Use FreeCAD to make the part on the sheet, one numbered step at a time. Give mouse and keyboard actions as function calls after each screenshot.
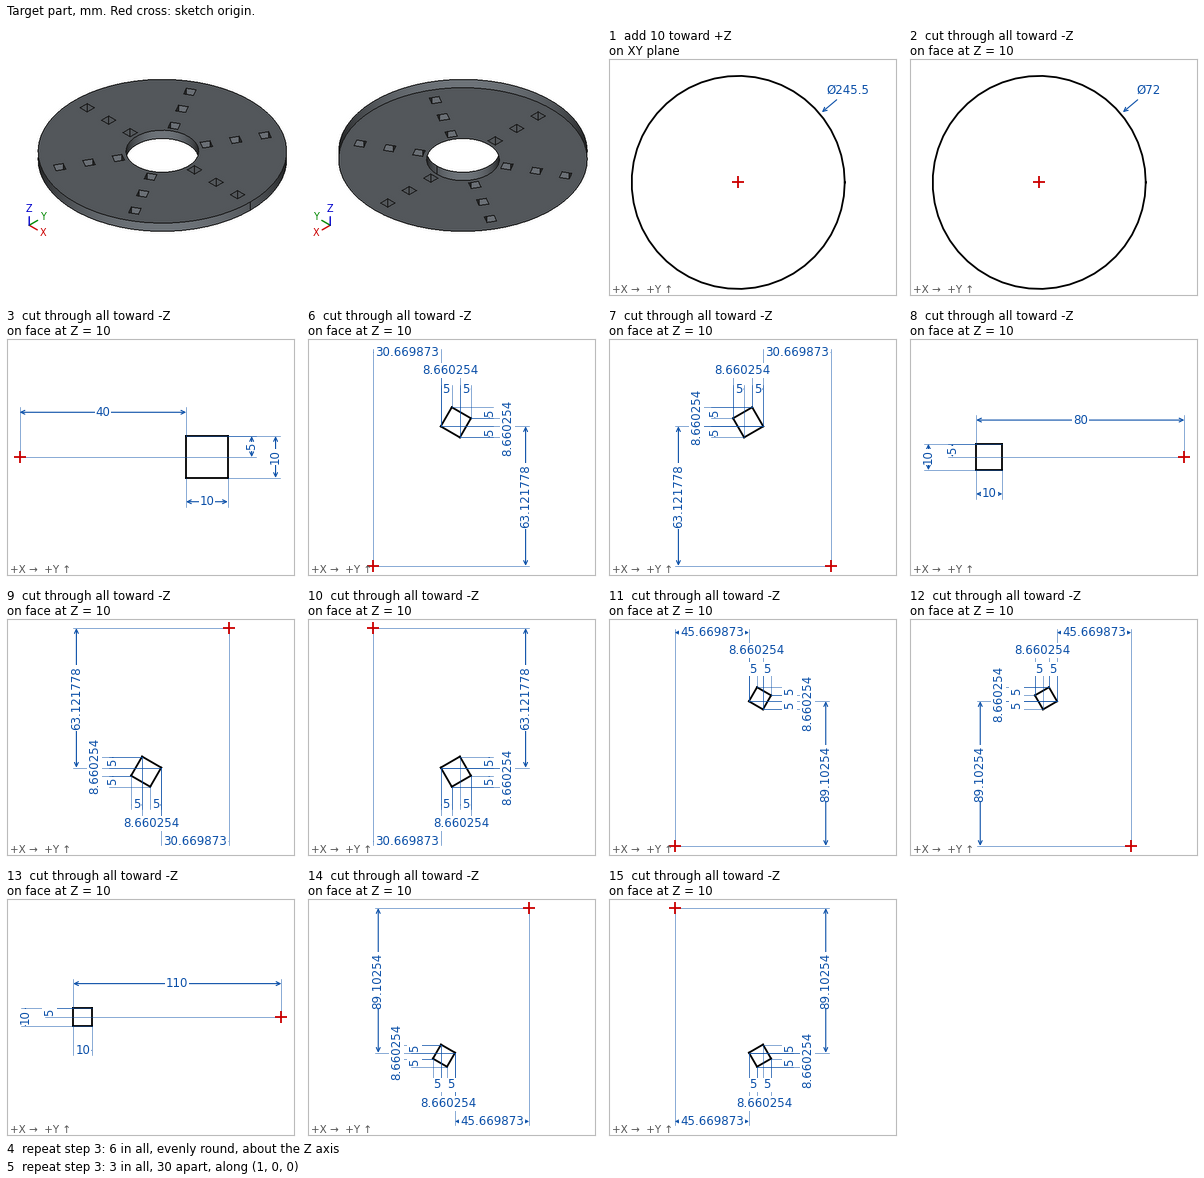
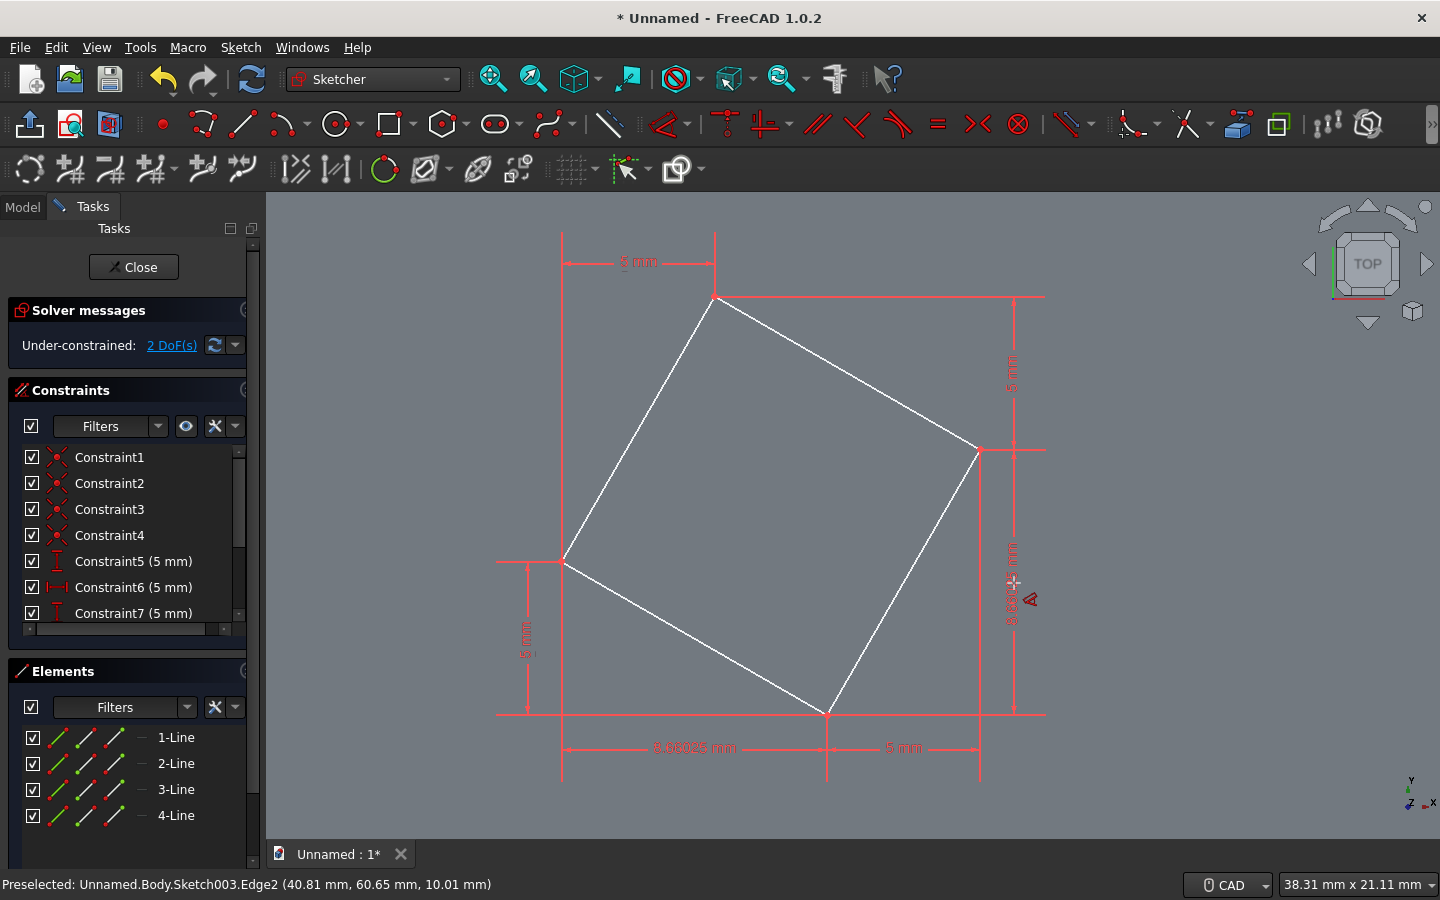
click(562, 562)
click(428, 528)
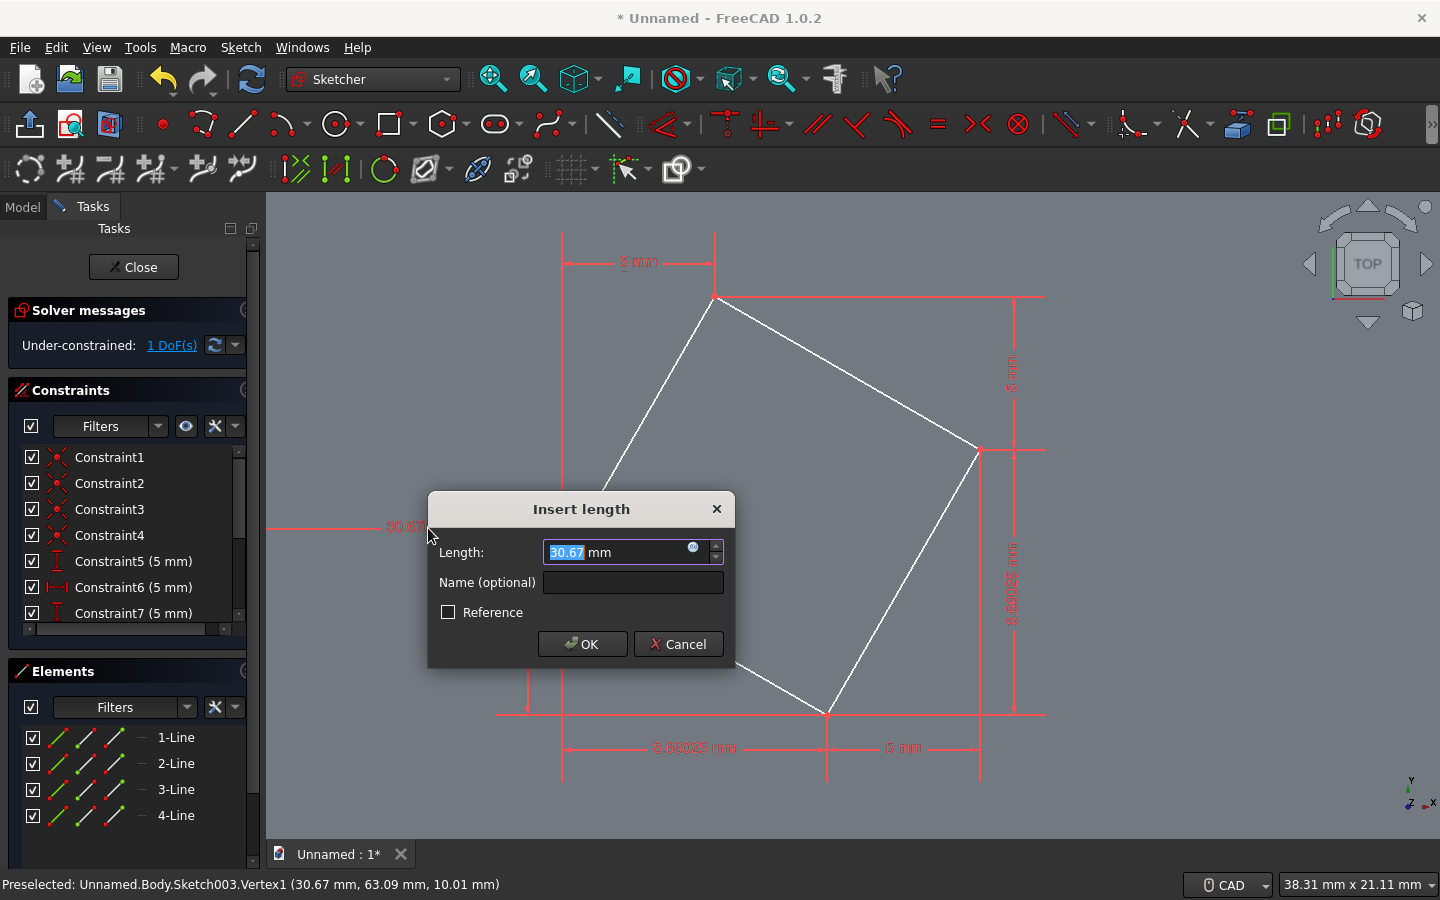
text(30.669873)
key(Return)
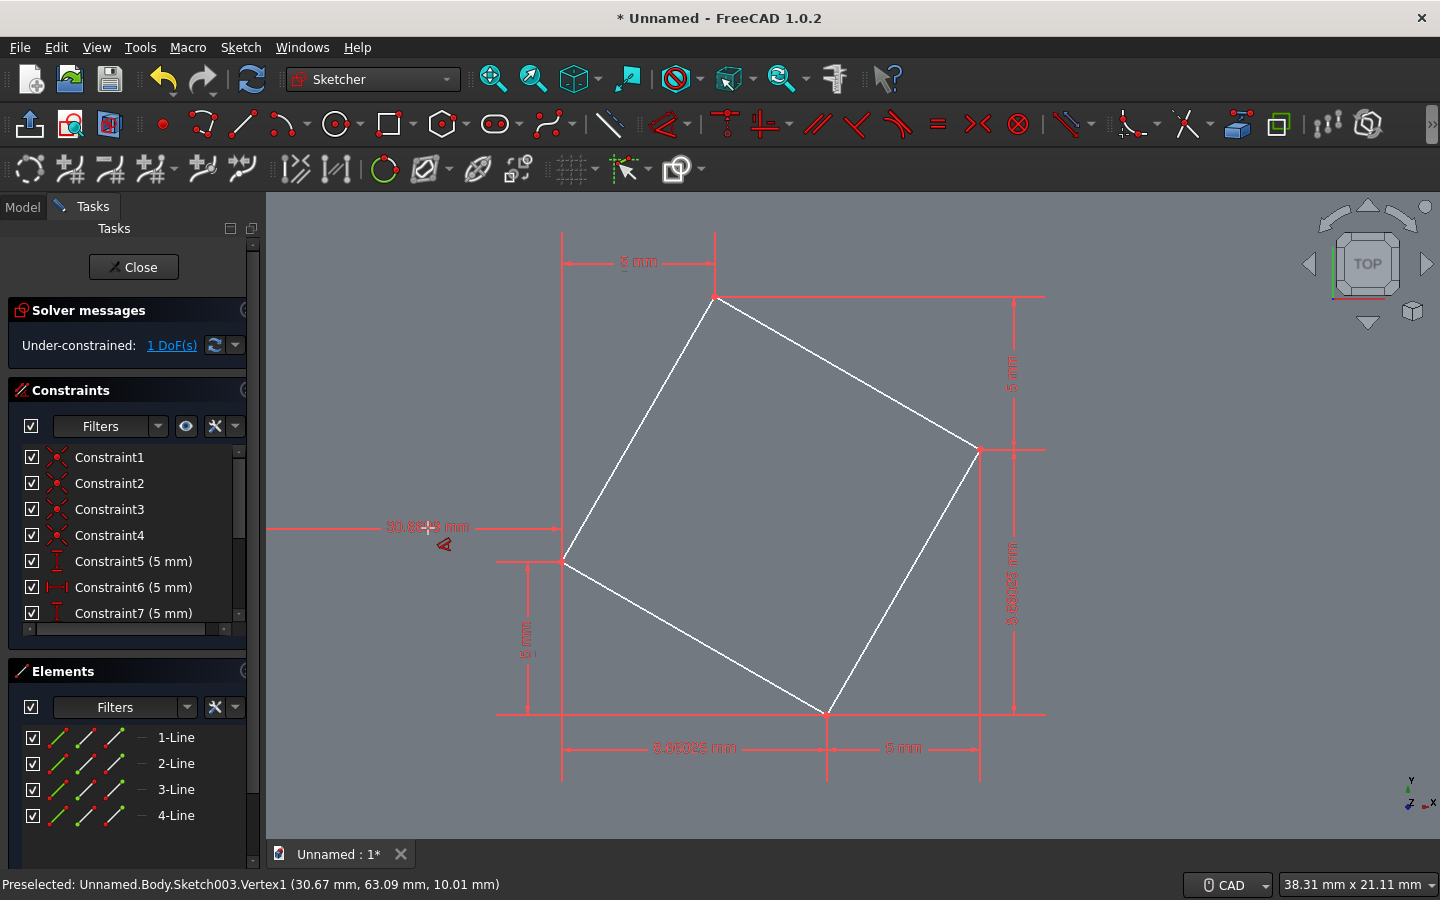
click(562, 562)
click(596, 687)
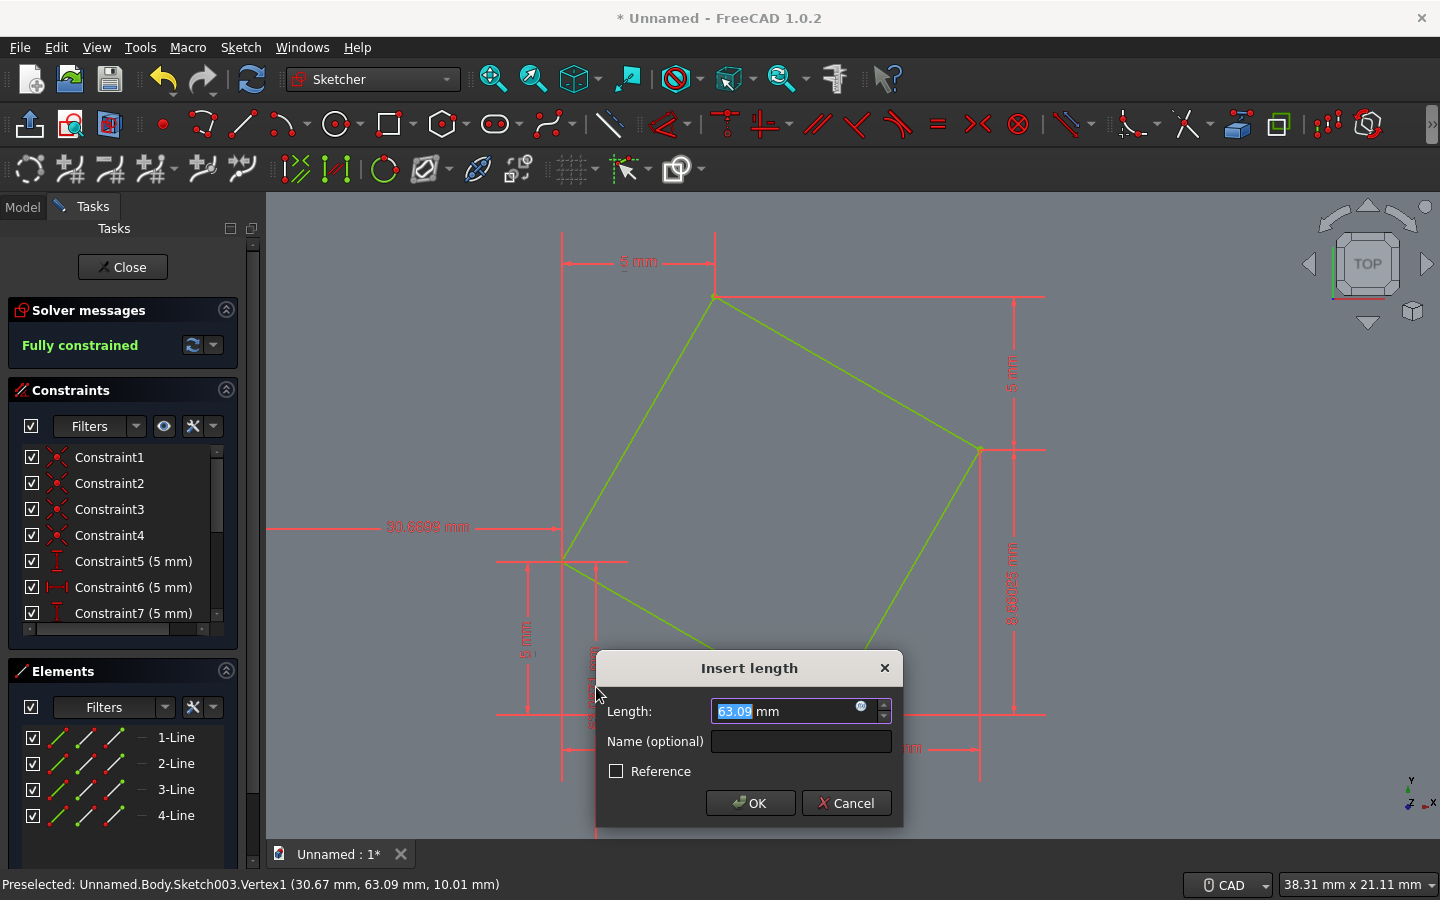
text(63.121778)
key(Return)
key(Escape)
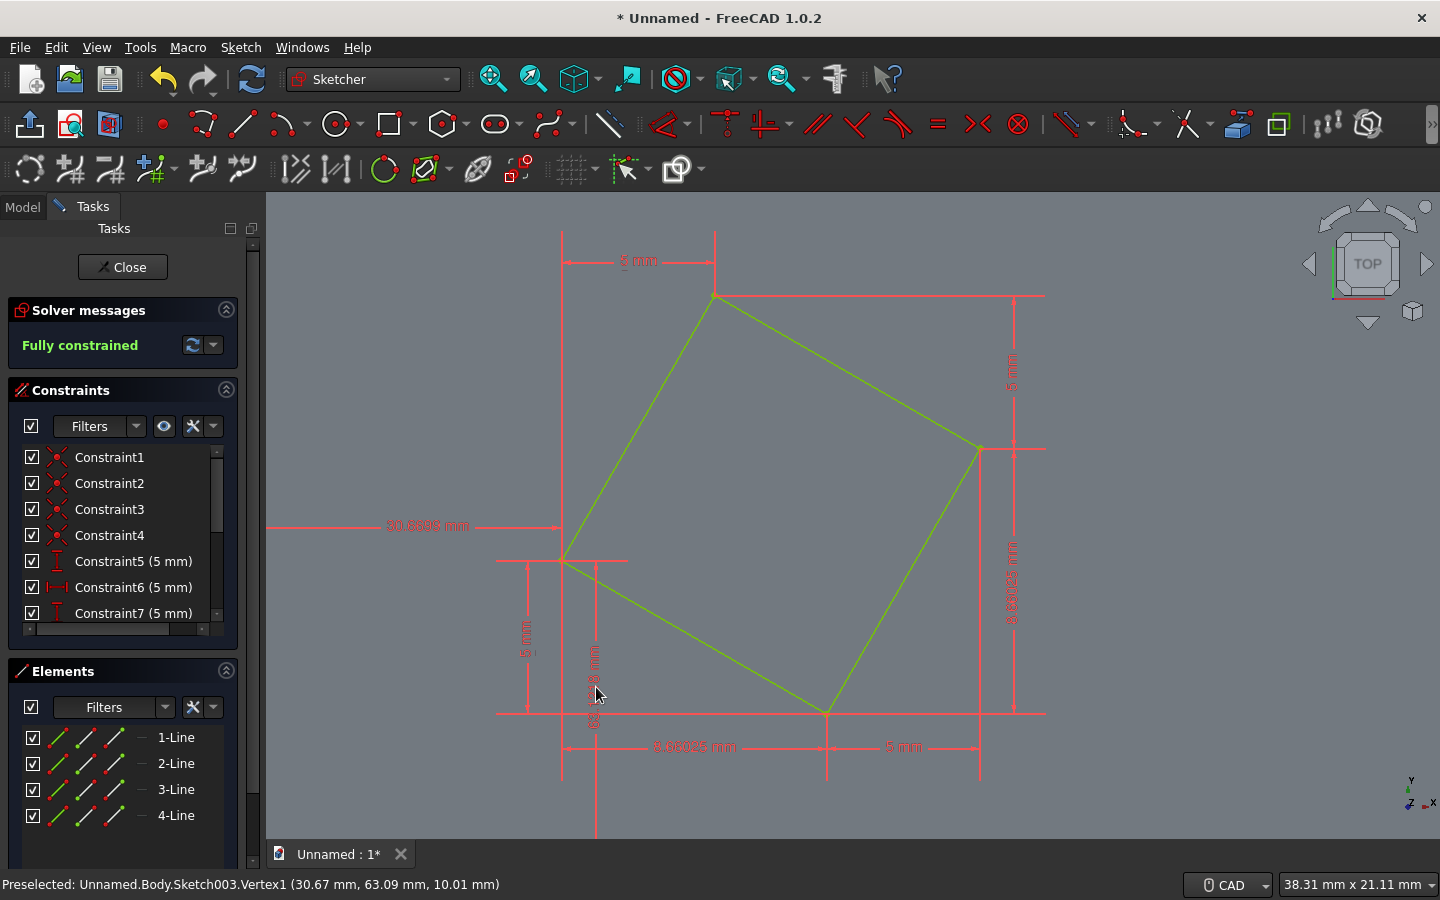
click(123, 267)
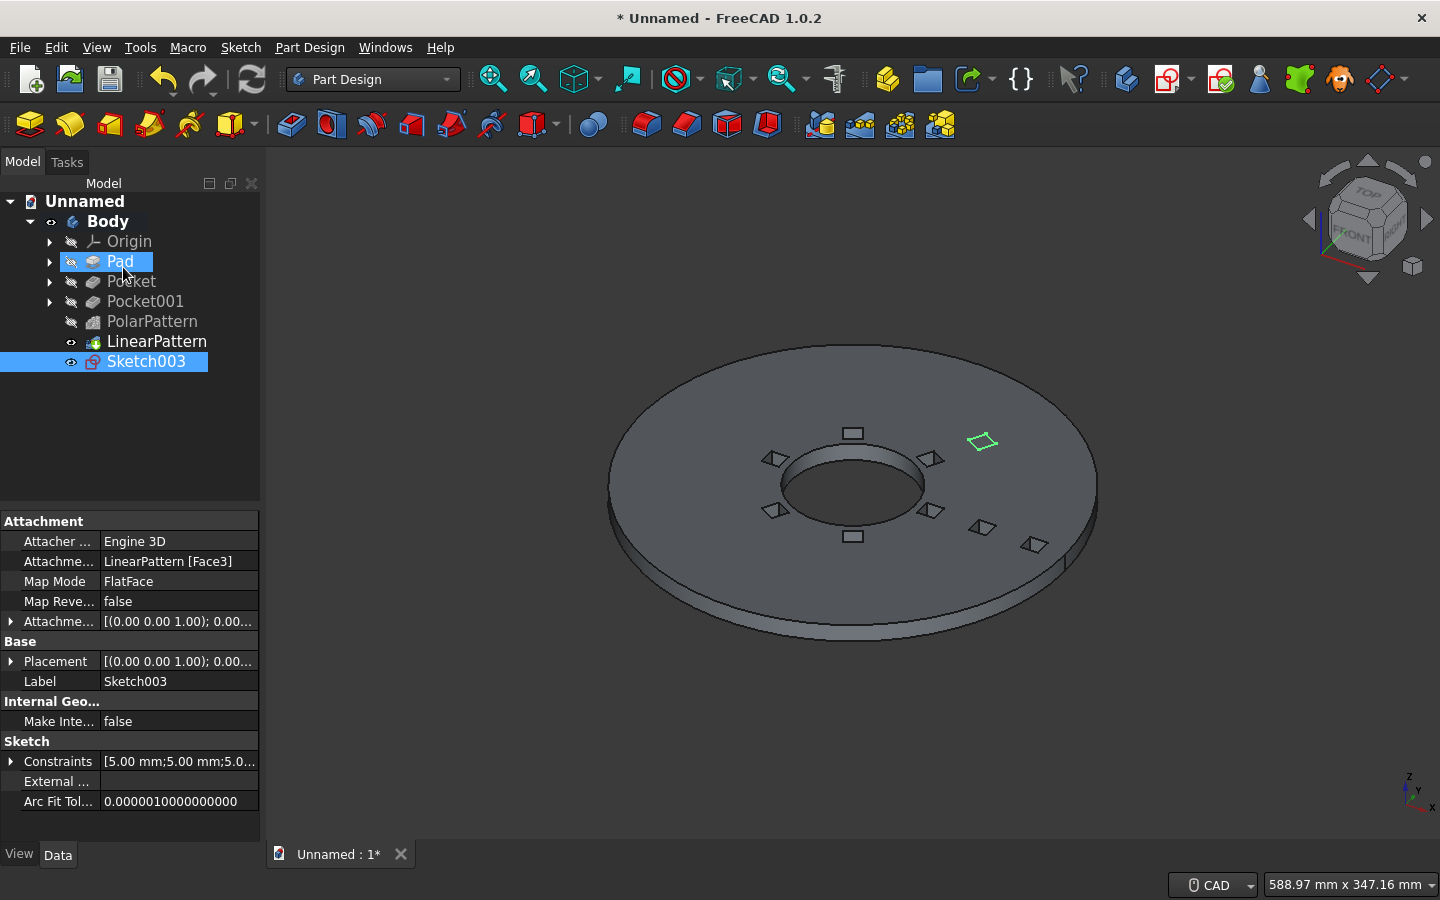
click(292, 124)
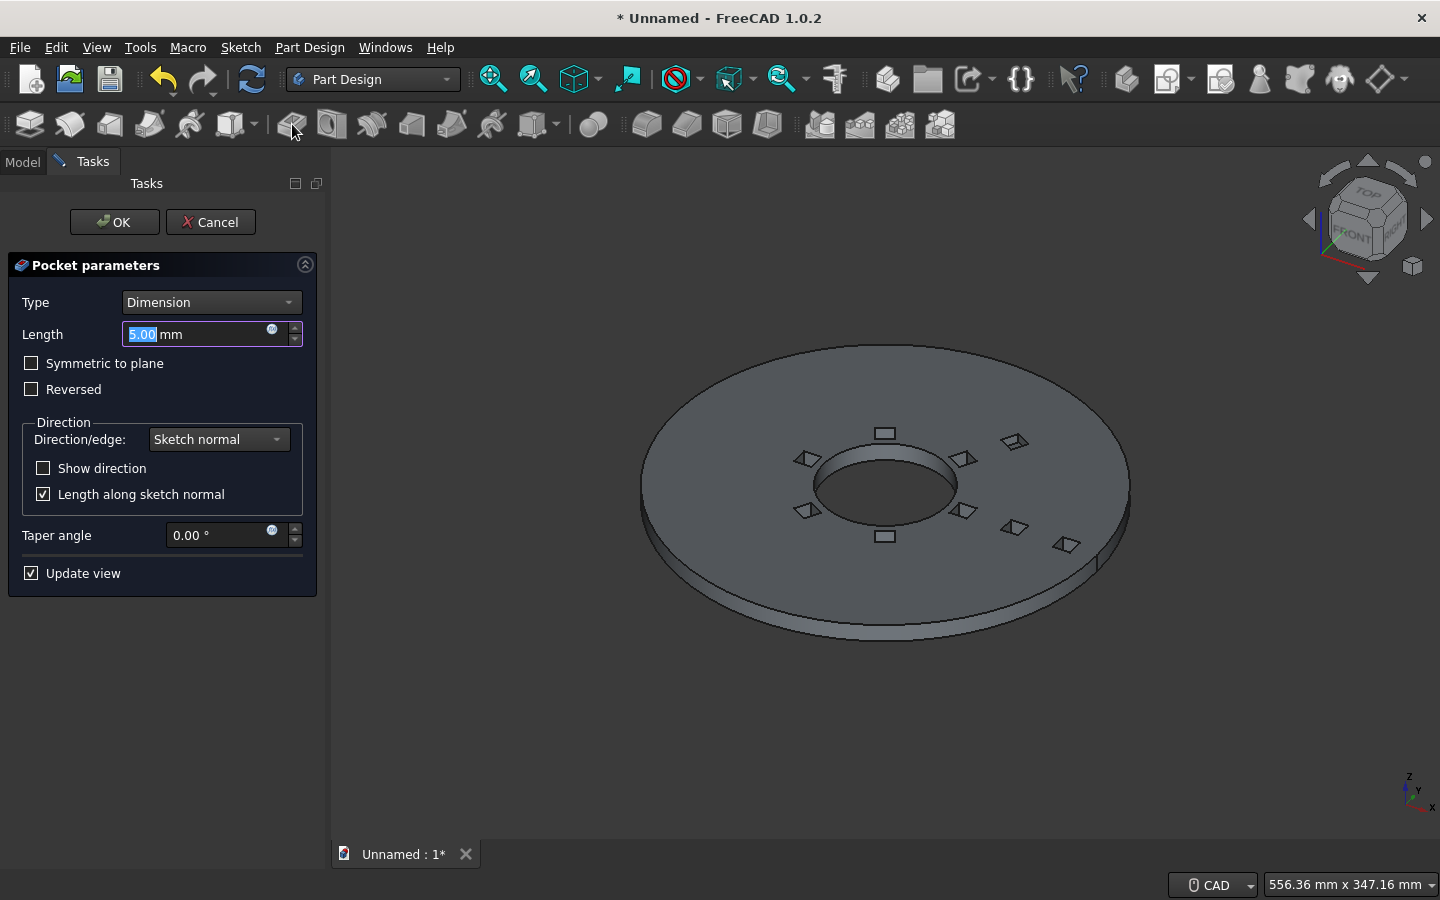
click(212, 302)